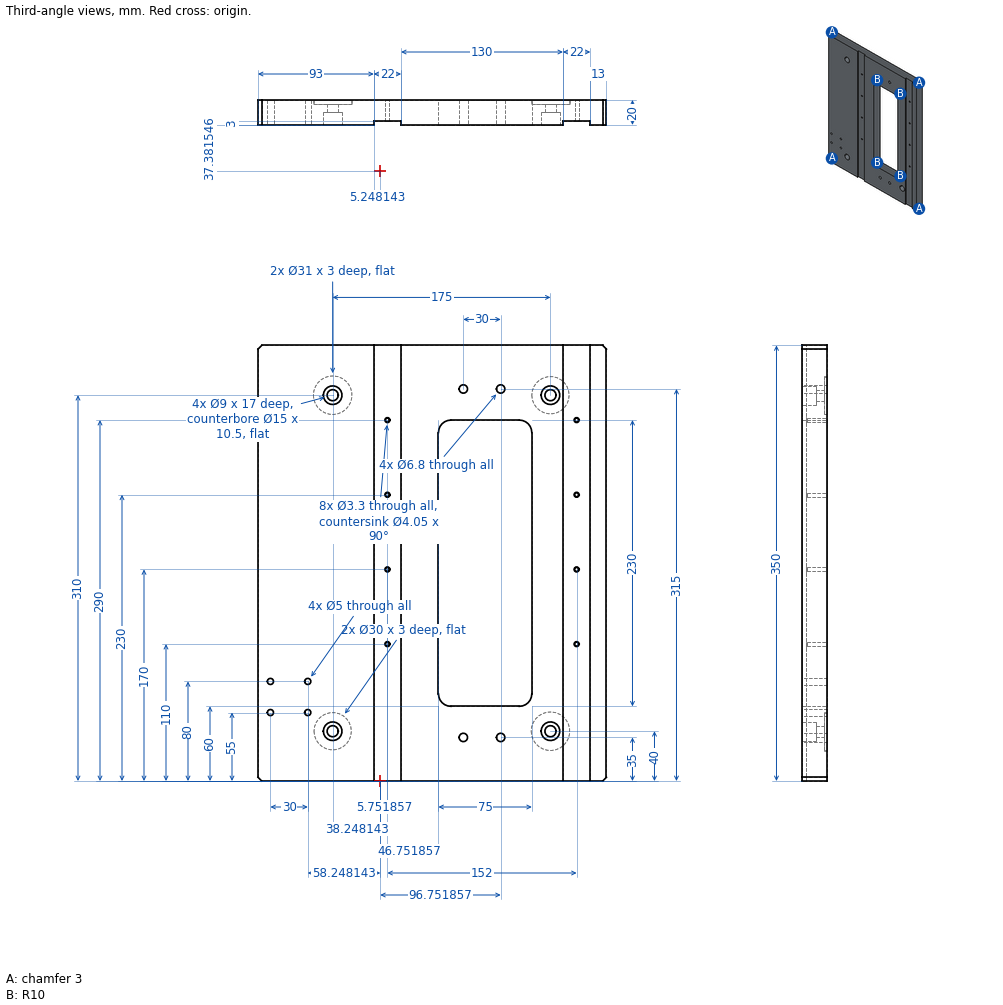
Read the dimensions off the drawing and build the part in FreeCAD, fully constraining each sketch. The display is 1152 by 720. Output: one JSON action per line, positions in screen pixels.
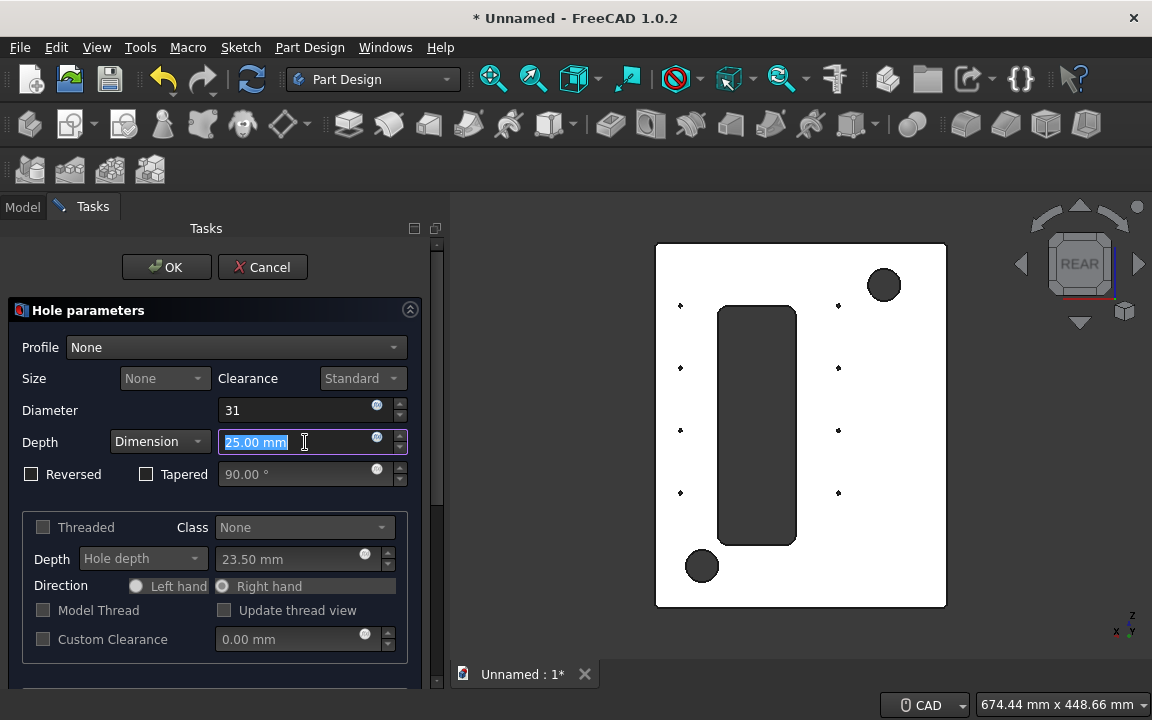
{"action": "type", "text": "3"}
{"action": "key", "text": "Tab"}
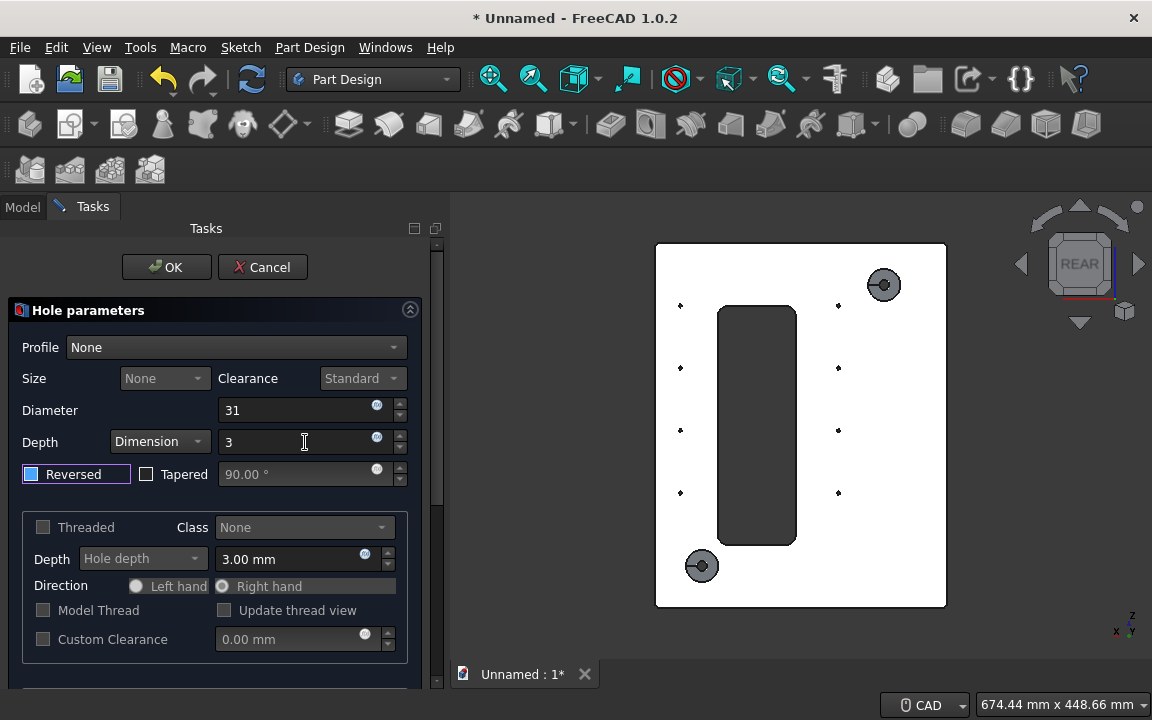
{"action": "scroll", "coordinate": [437, 463], "scroll_direction": "down", "scroll_amount": 5}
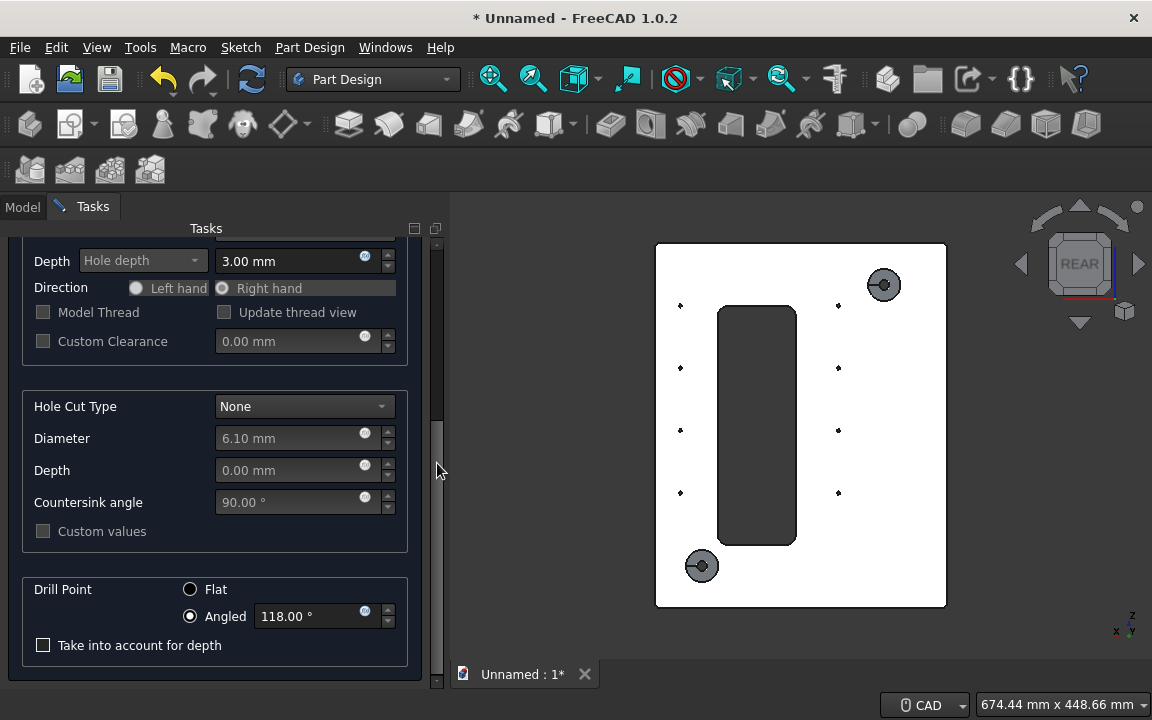
{"action": "left_click", "coordinate": [191, 589]}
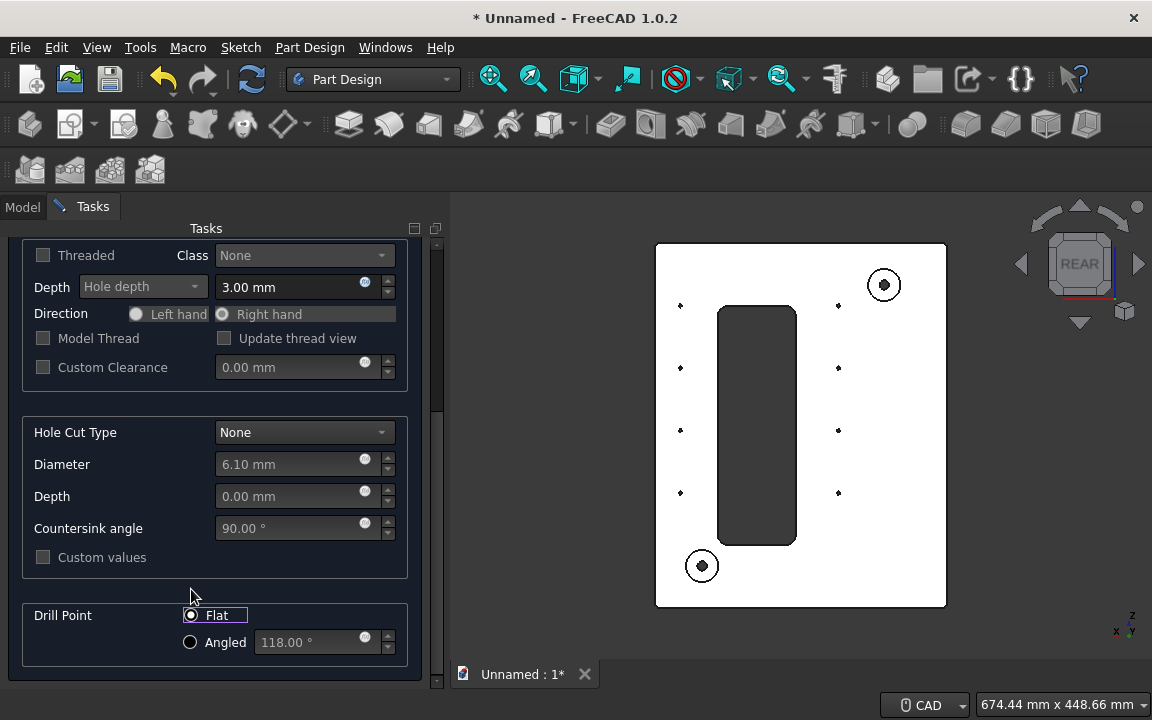
{"action": "scroll", "coordinate": [437, 463], "scroll_direction": "up", "scroll_amount": 6}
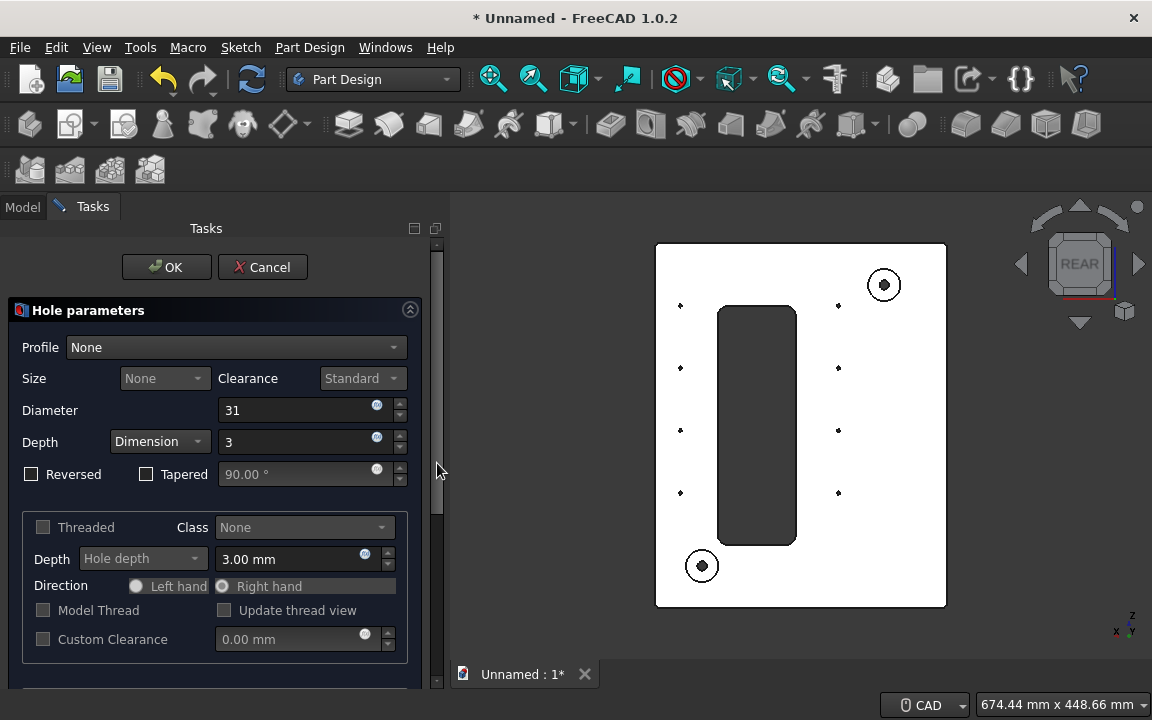
{"action": "left_click", "coordinate": [167, 267]}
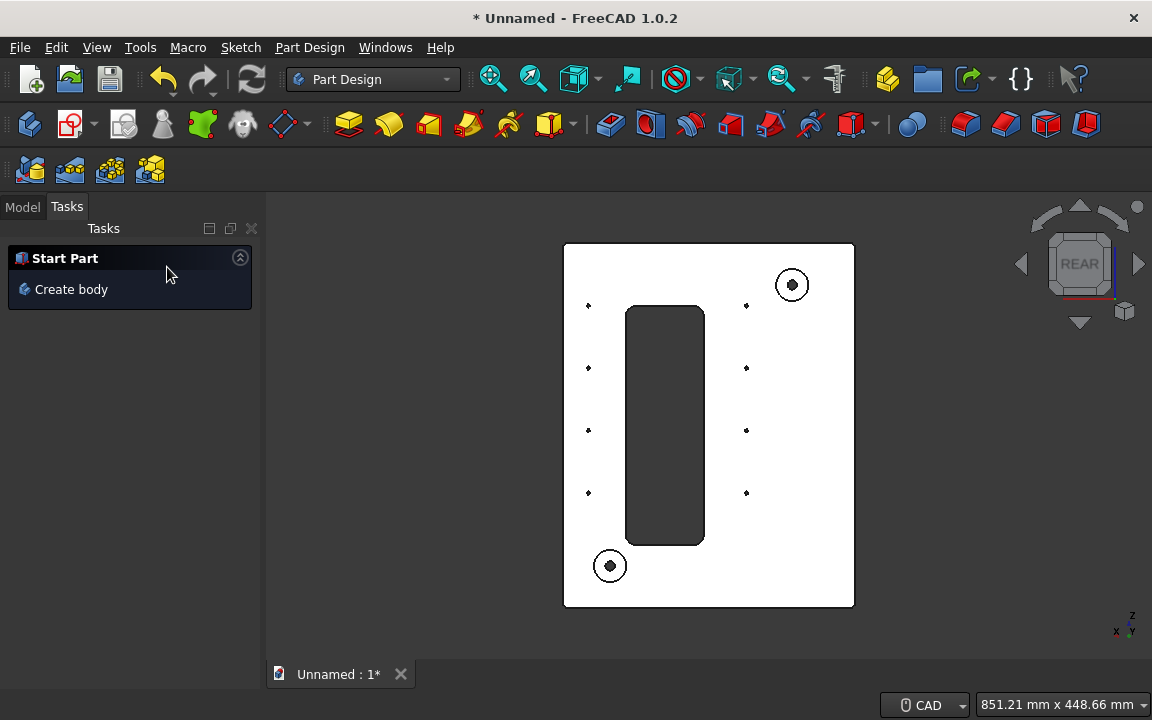
{"action": "left_click", "coordinate": [792, 529]}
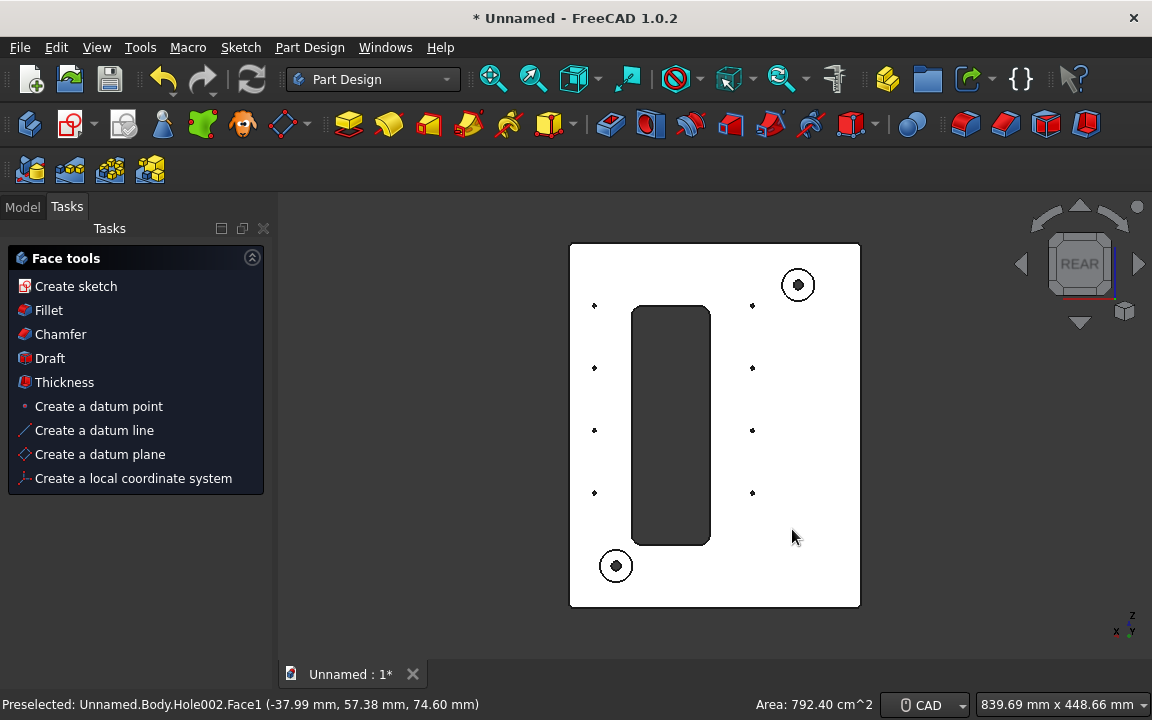
{"action": "left_click", "coordinate": [70, 124]}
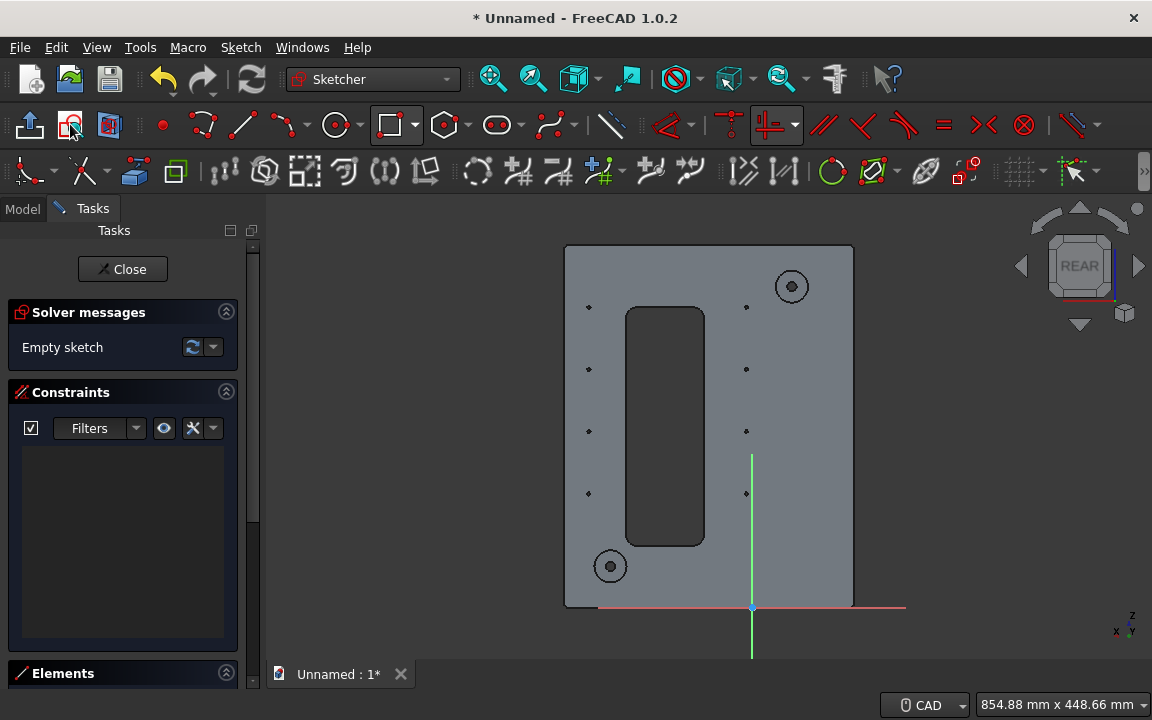
{"action": "scroll", "coordinate": [366, 368], "scroll_direction": "down", "scroll_amount": 1}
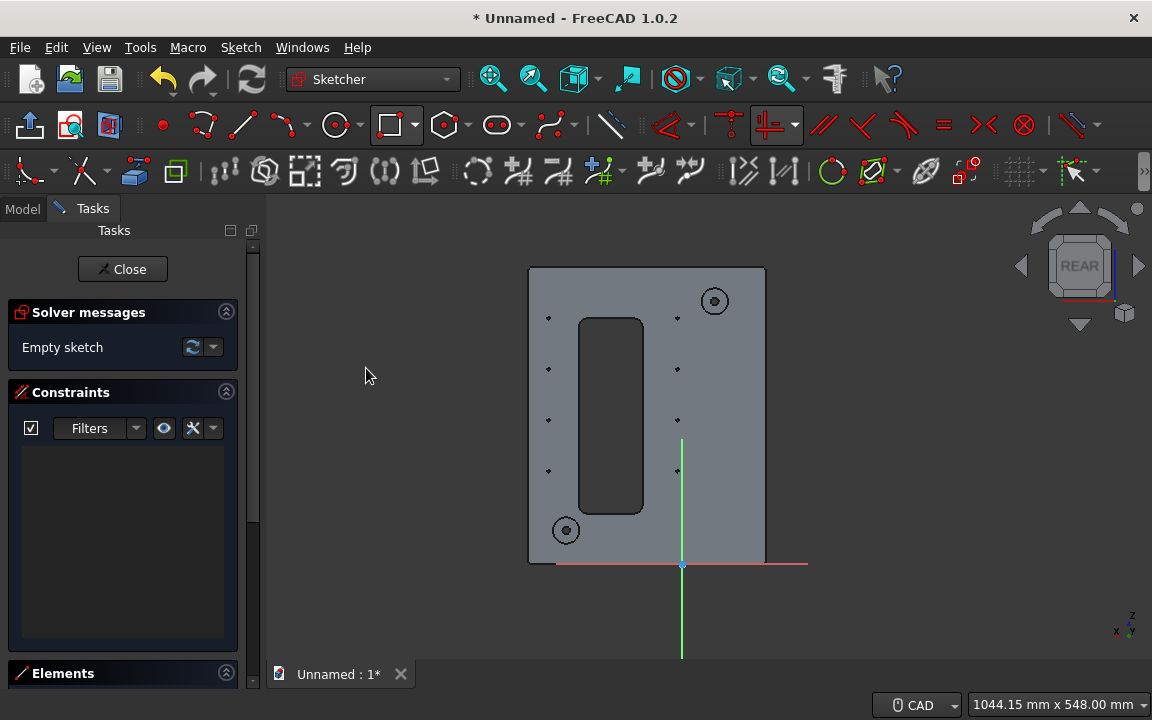
{"action": "left_click", "coordinate": [336, 126]}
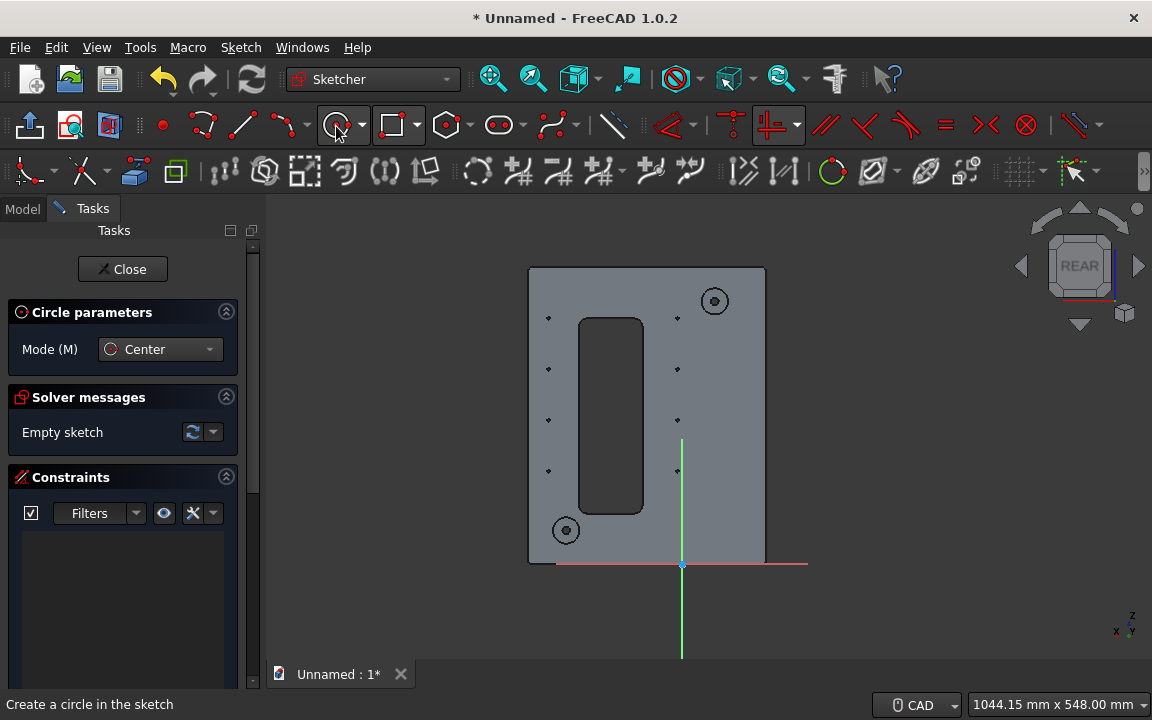
{"action": "scroll", "coordinate": [715, 531], "scroll_direction": "up", "scroll_amount": 3}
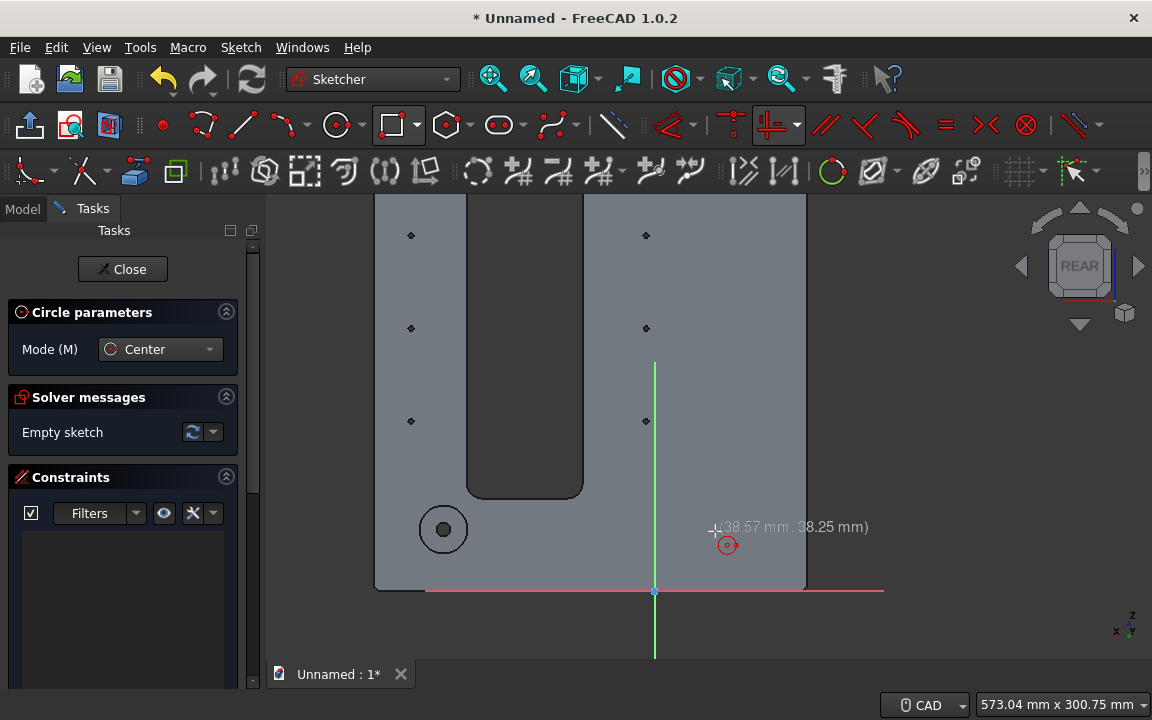
{"action": "left_click", "coordinate": [714, 530]}
{"action": "mouse_move", "coordinate": [730, 513]}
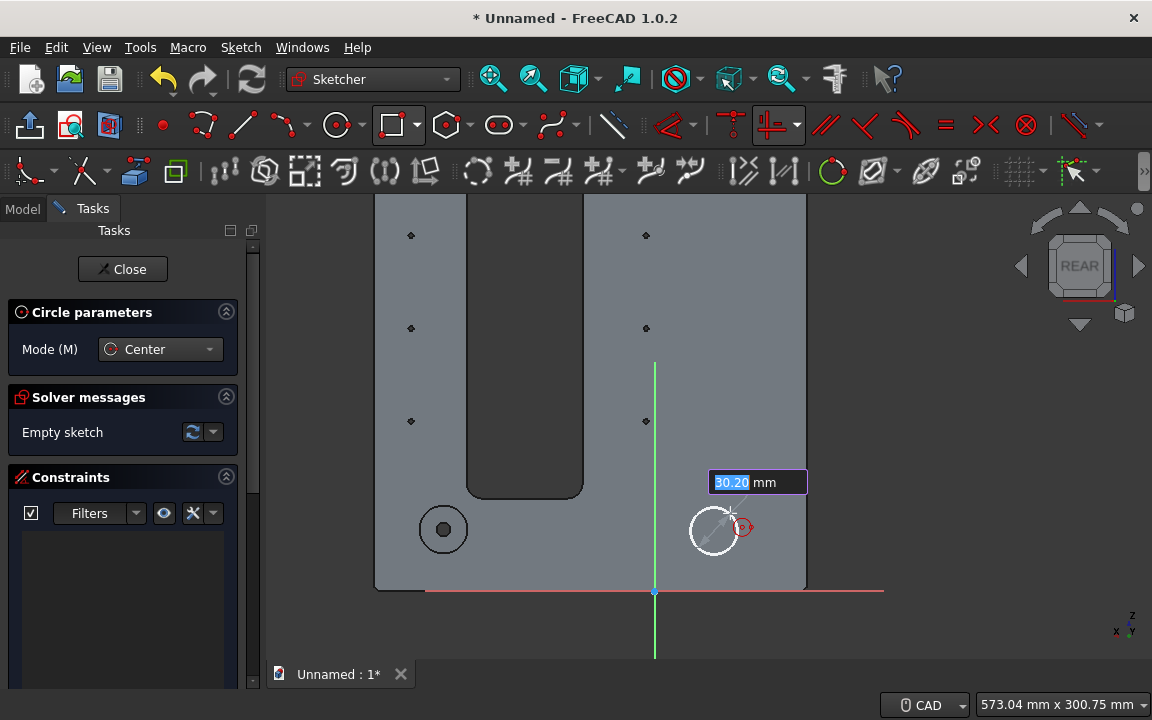
{"action": "type", "text": "30"}
{"action": "key", "text": "Return"}